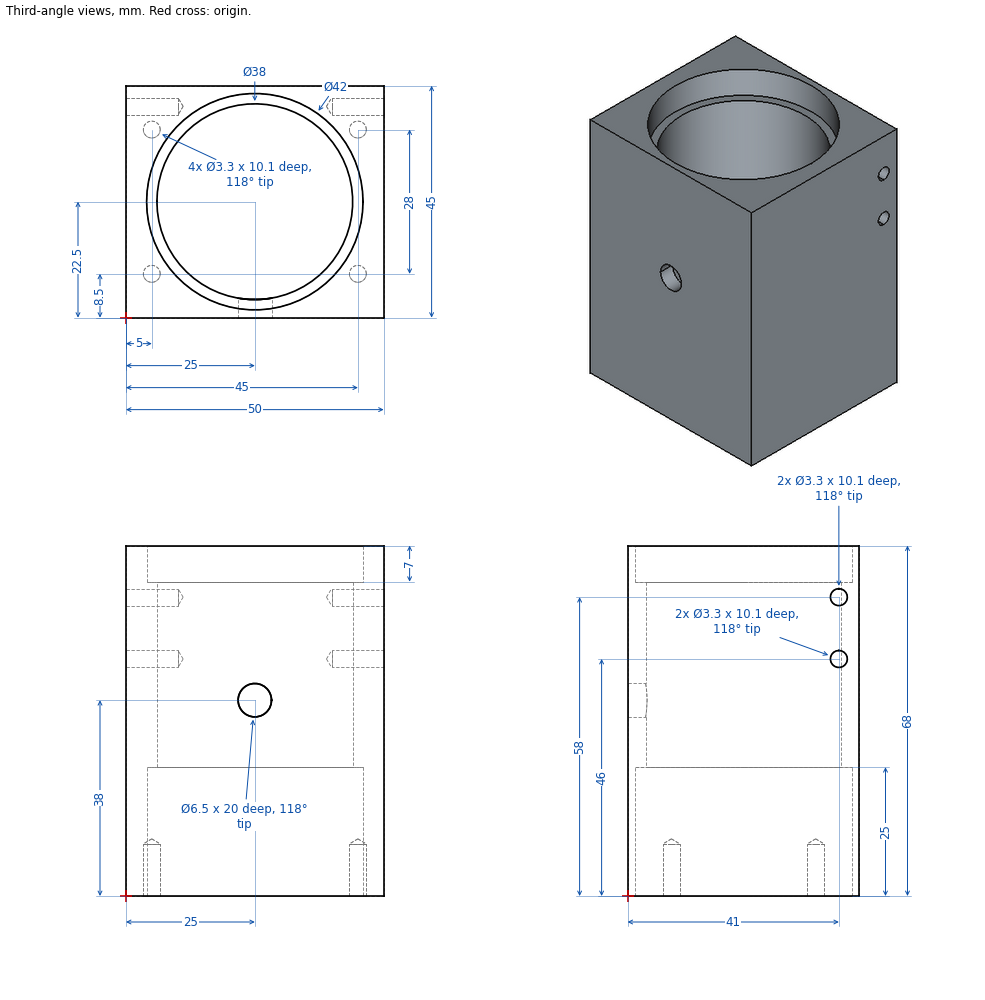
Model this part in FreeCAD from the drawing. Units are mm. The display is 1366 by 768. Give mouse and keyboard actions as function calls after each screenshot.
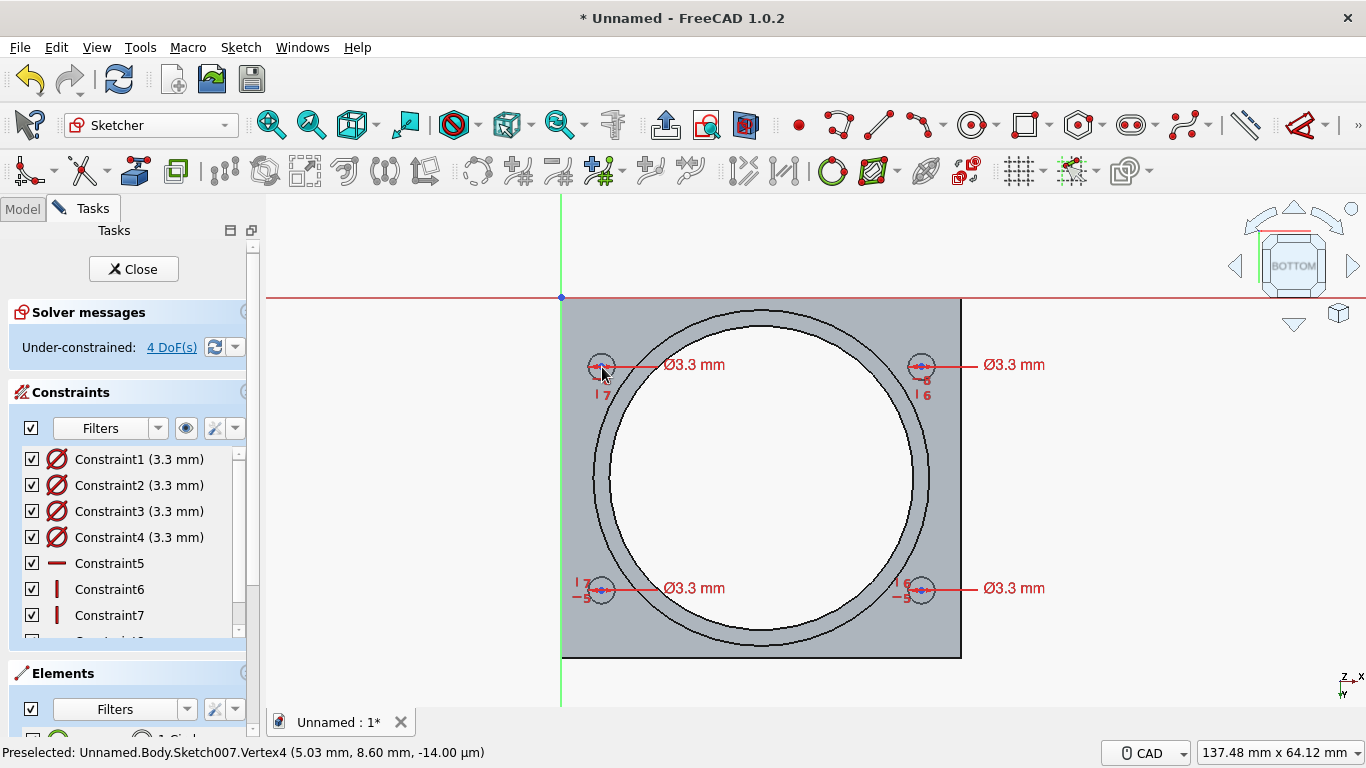
click(1300, 126)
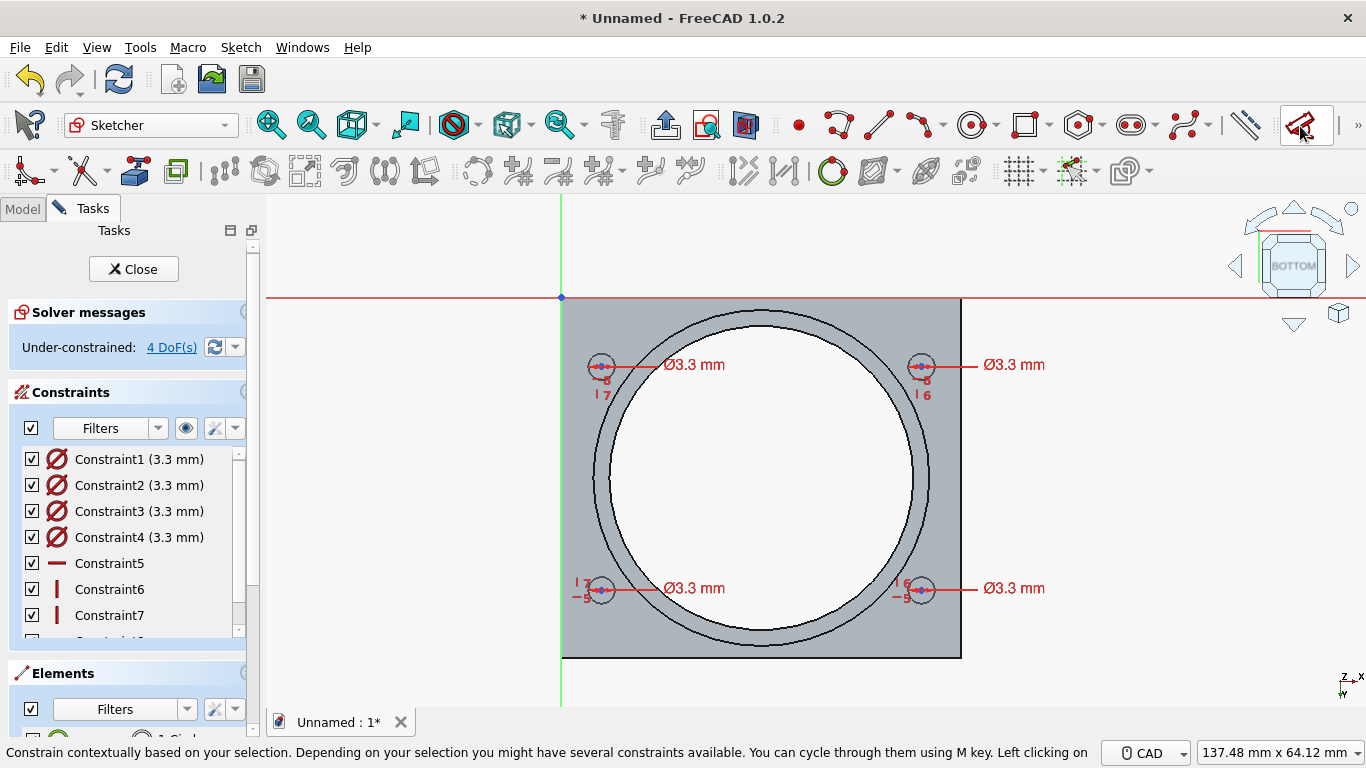
click(602, 590)
click(581, 264)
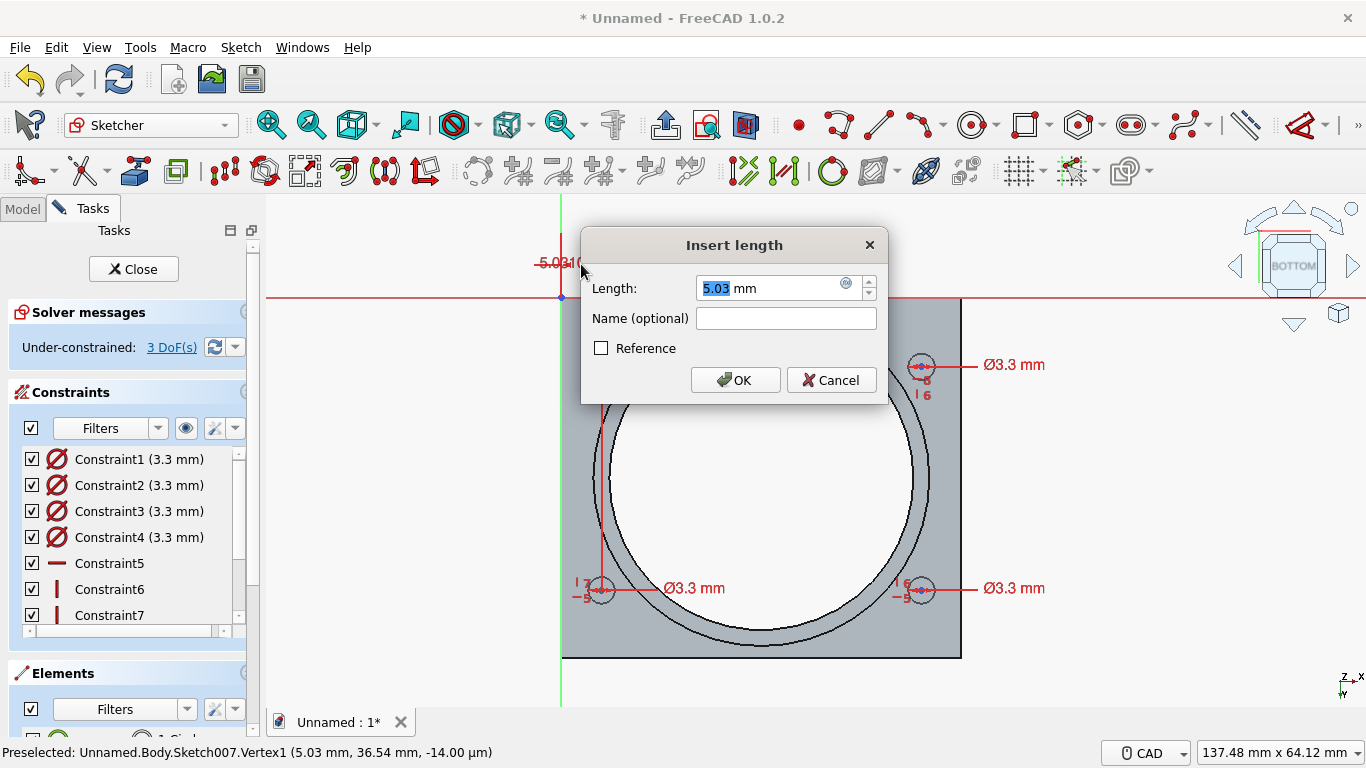
text(5)
key(Return)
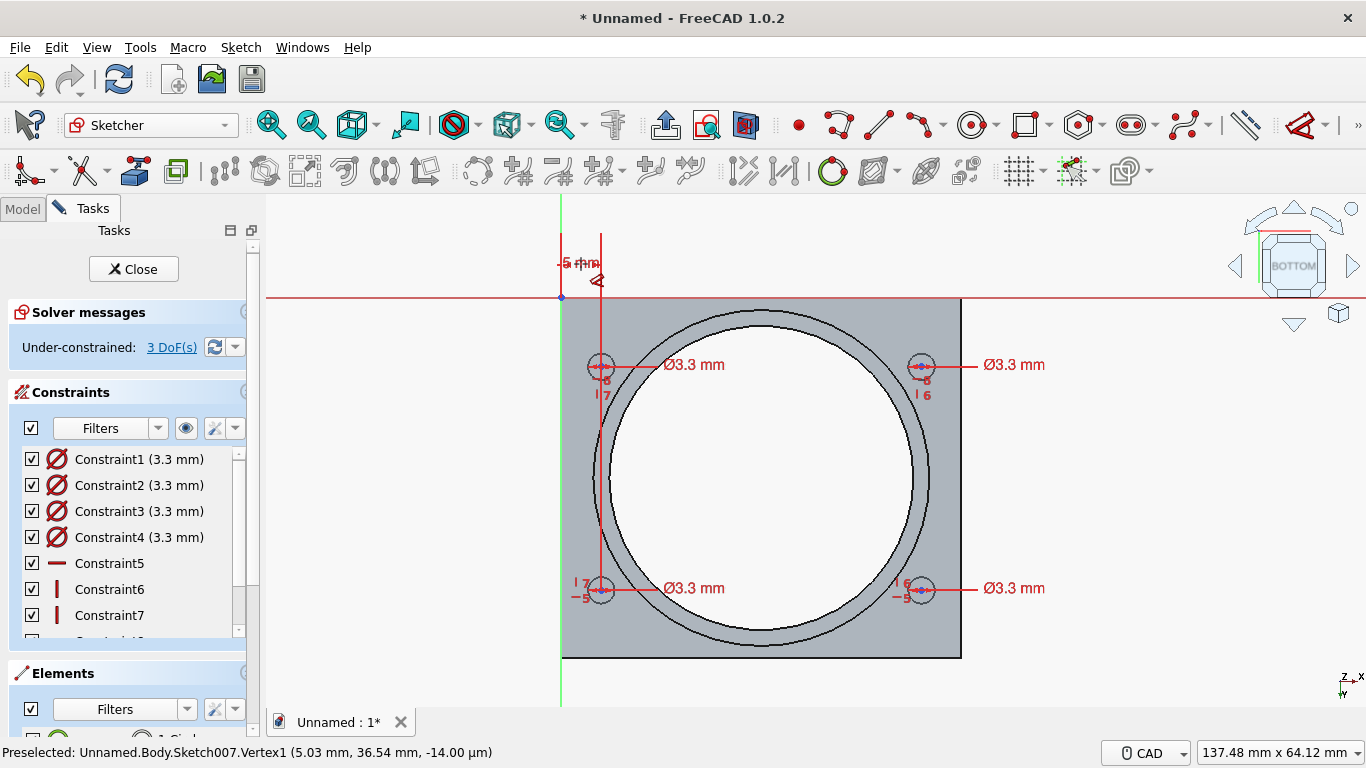
click(922, 590)
click(741, 264)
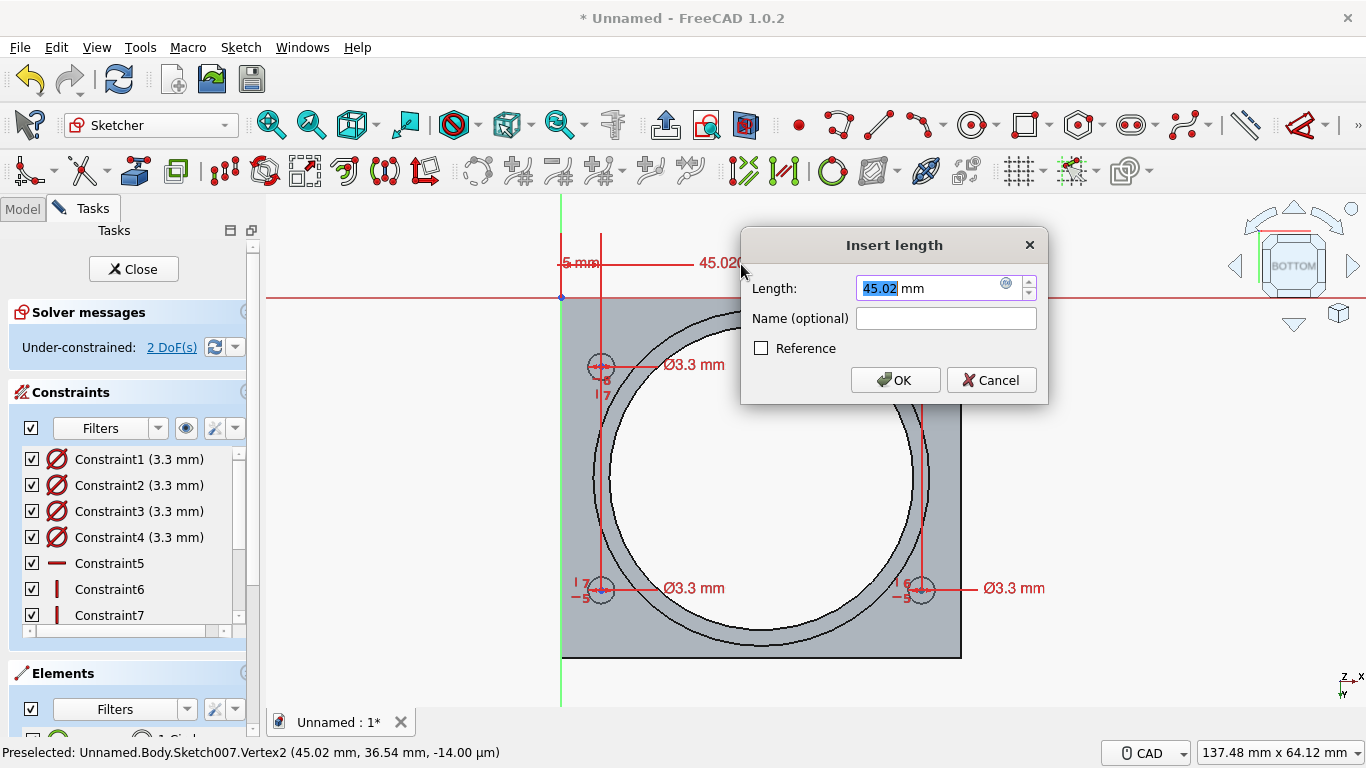
text(45)
key(Return)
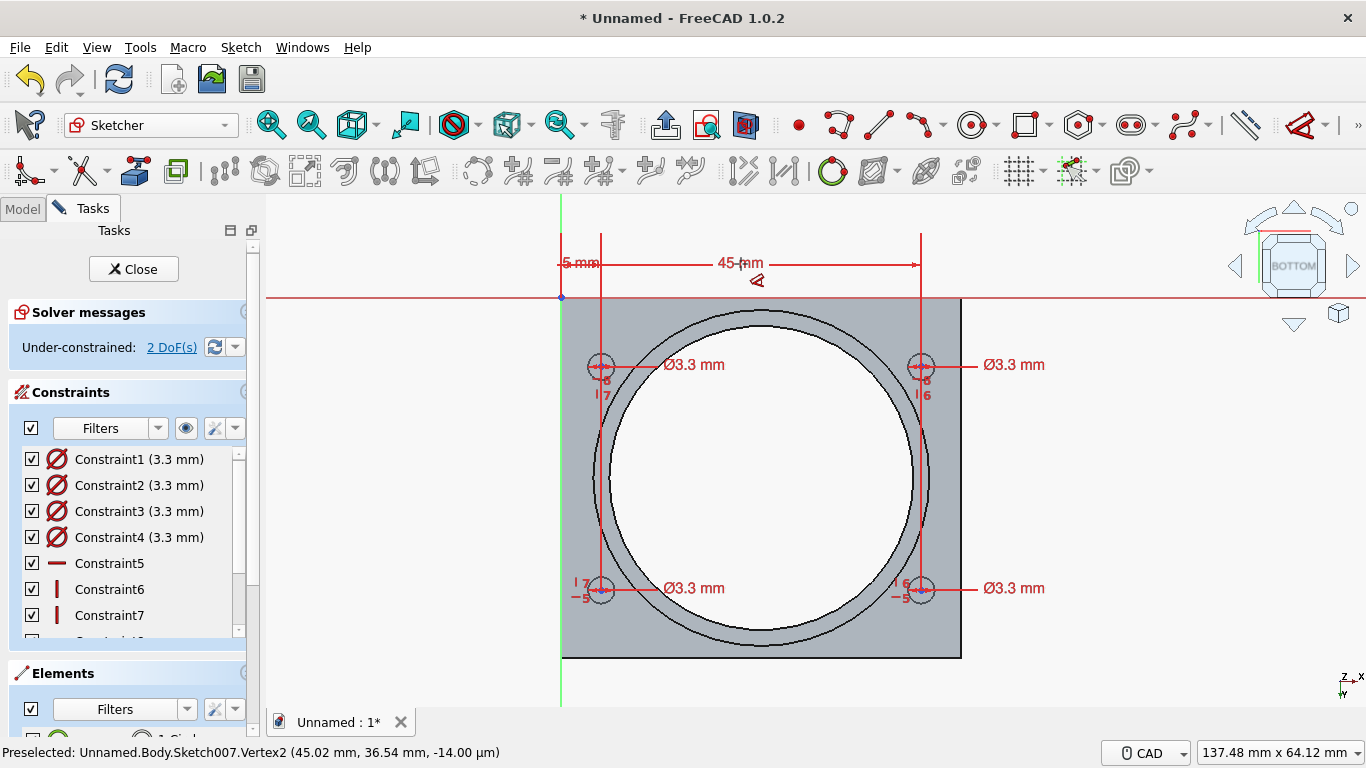
click(921, 367)
click(527, 332)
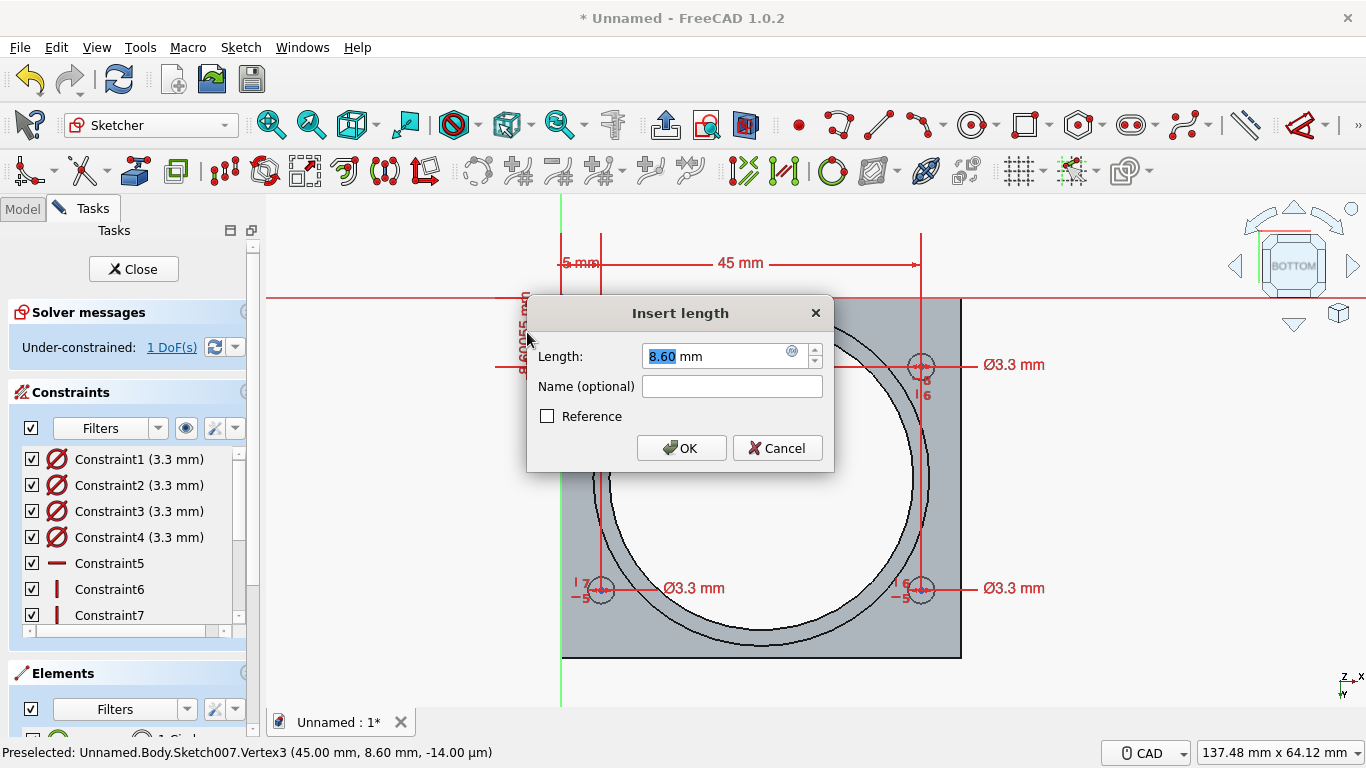
text(8.5)
key(Return)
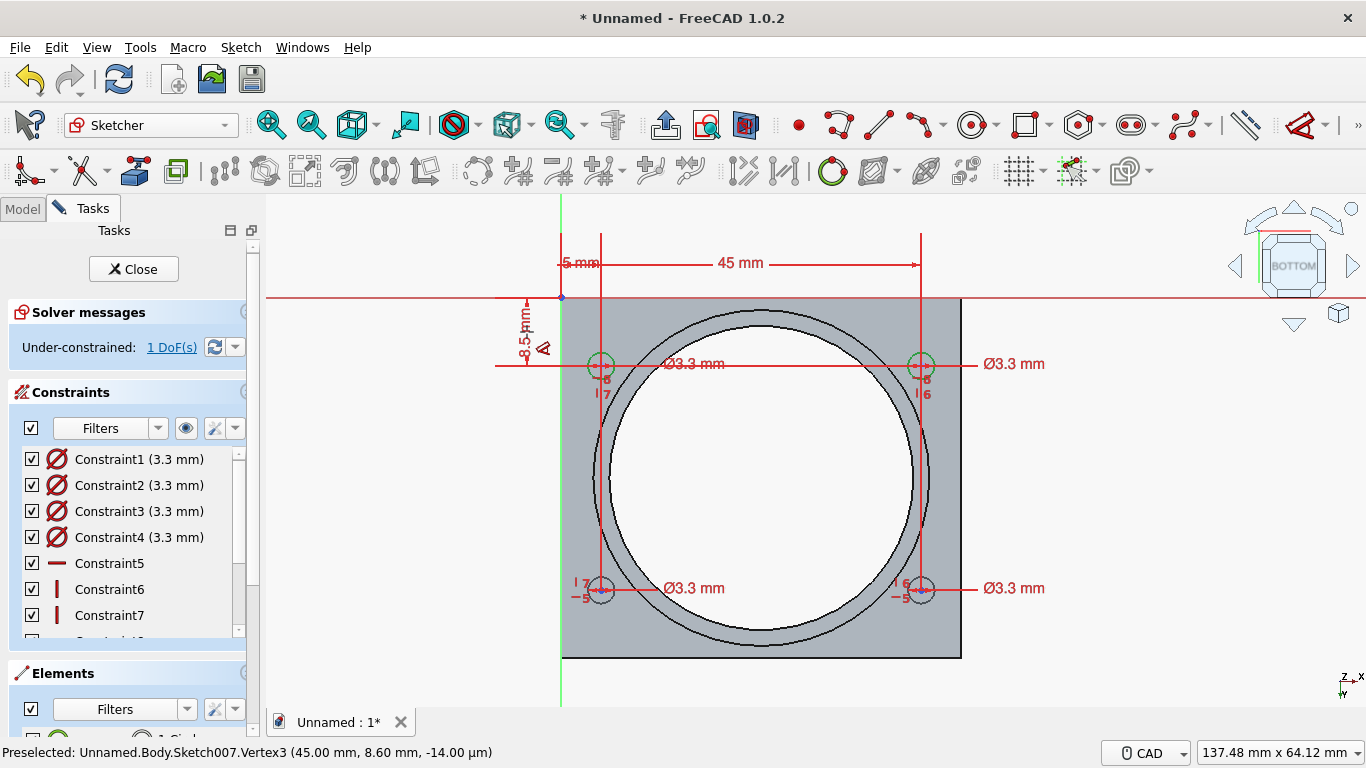
click(921, 590)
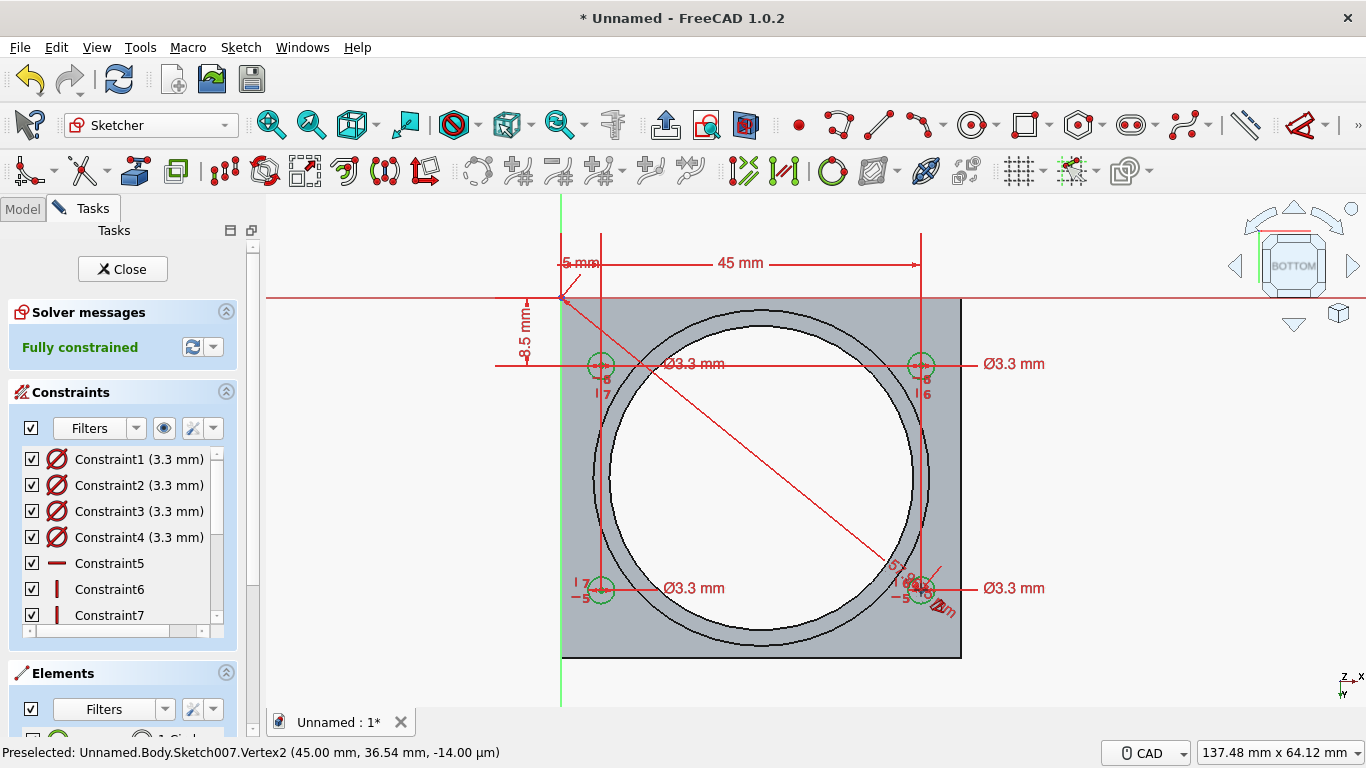
click(921, 366)
click(955, 478)